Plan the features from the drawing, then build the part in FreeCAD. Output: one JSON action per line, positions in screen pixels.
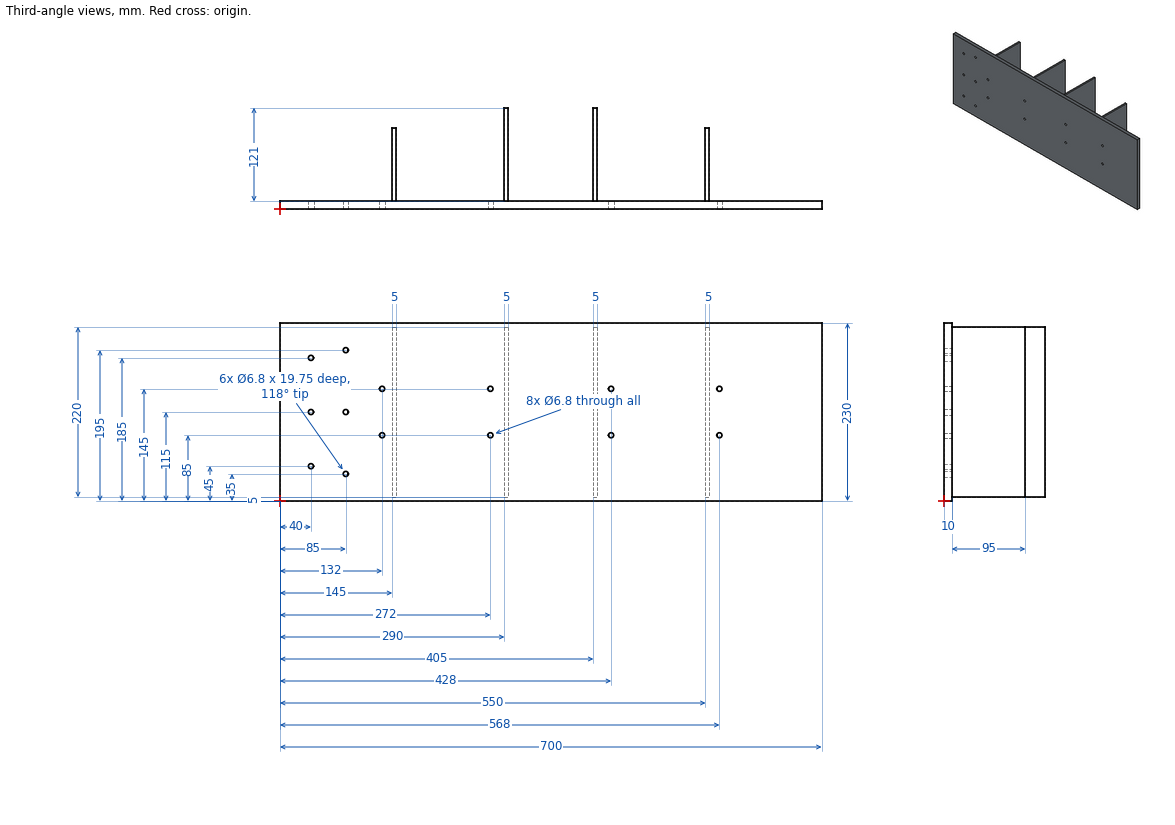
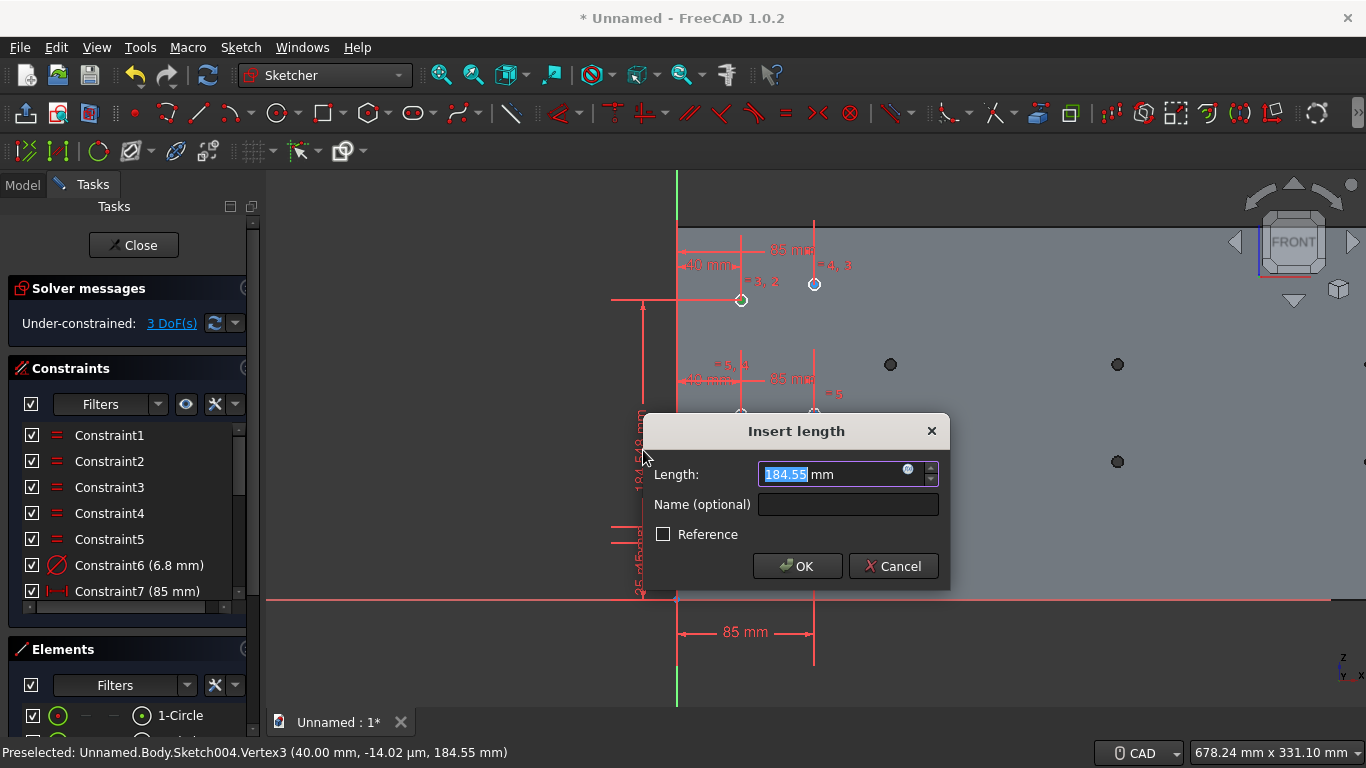
{"action": "type", "text": "185"}
{"action": "key", "text": "Return"}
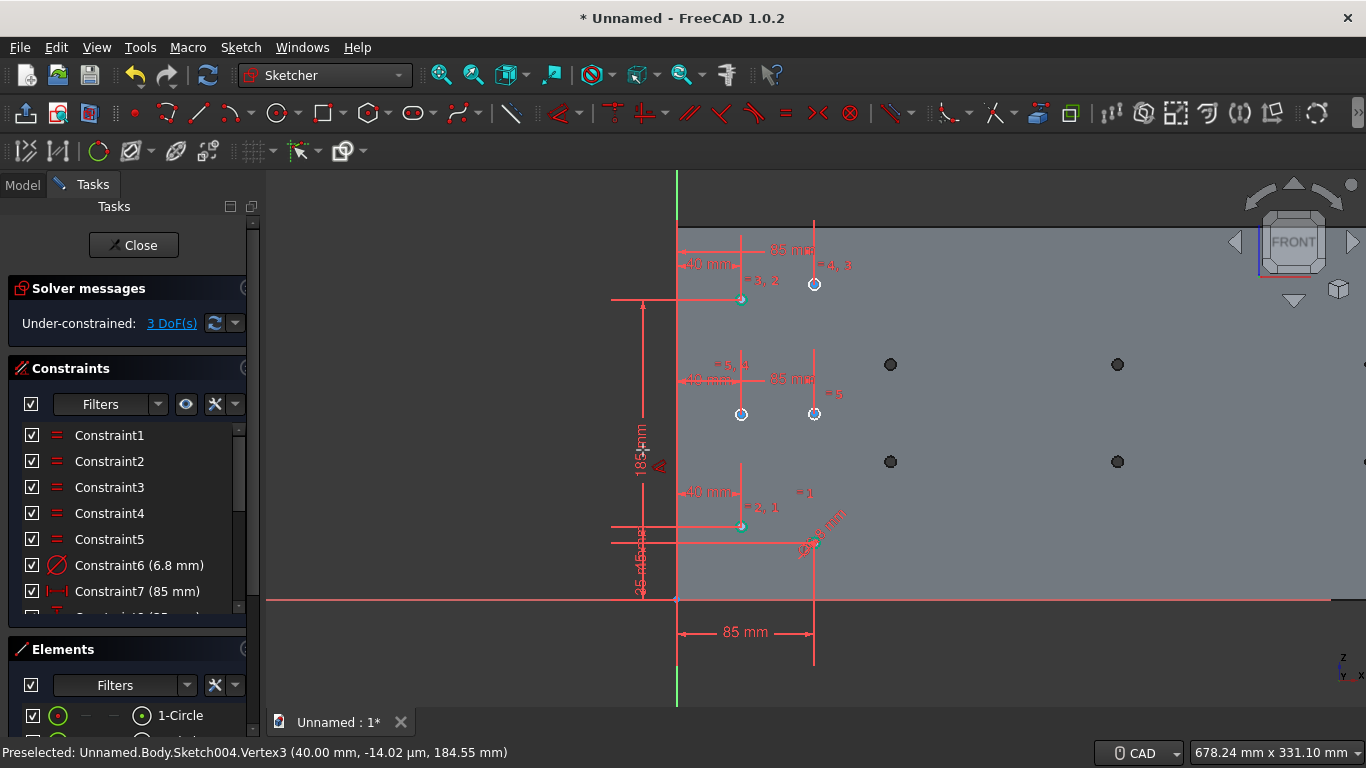
{"action": "left_click", "coordinate": [814, 285]}
{"action": "left_click", "coordinate": [643, 515]}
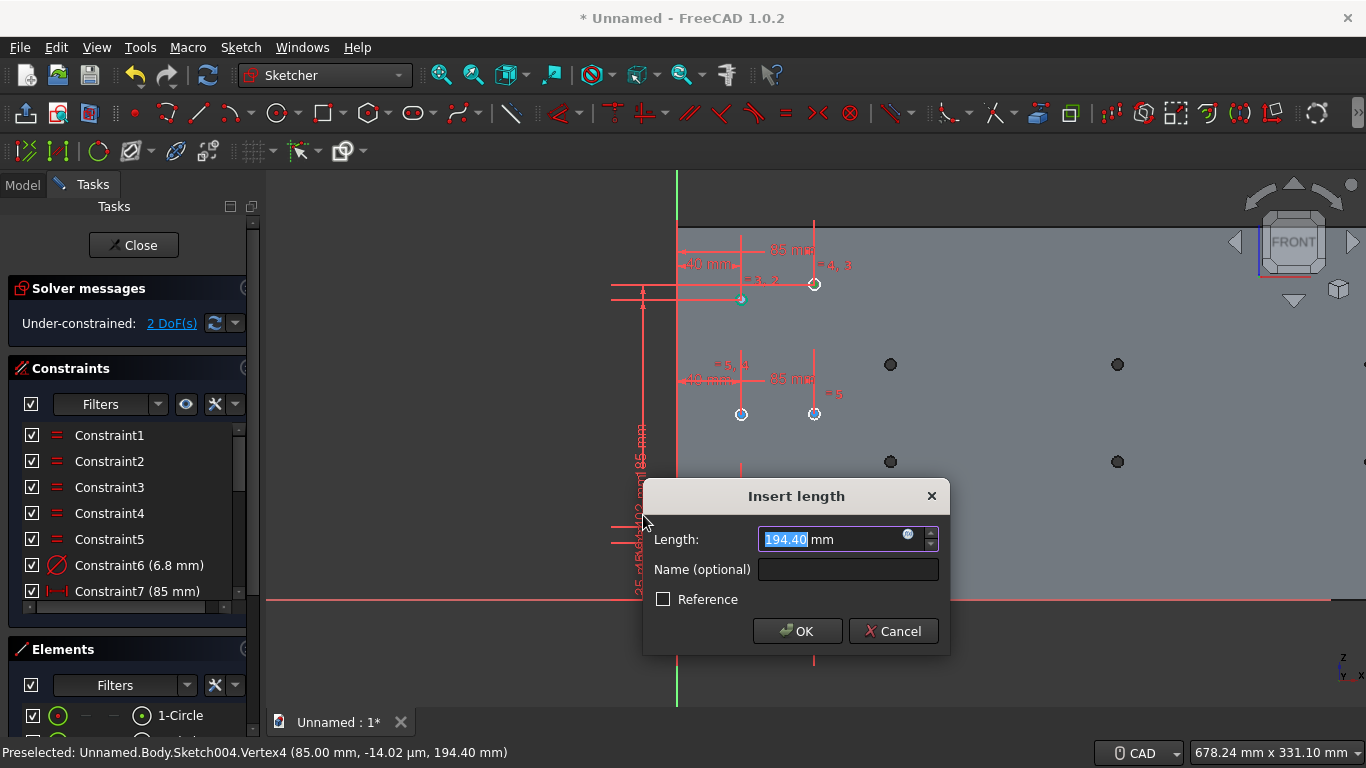
{"action": "type", "text": "195"}
{"action": "key", "text": "Return"}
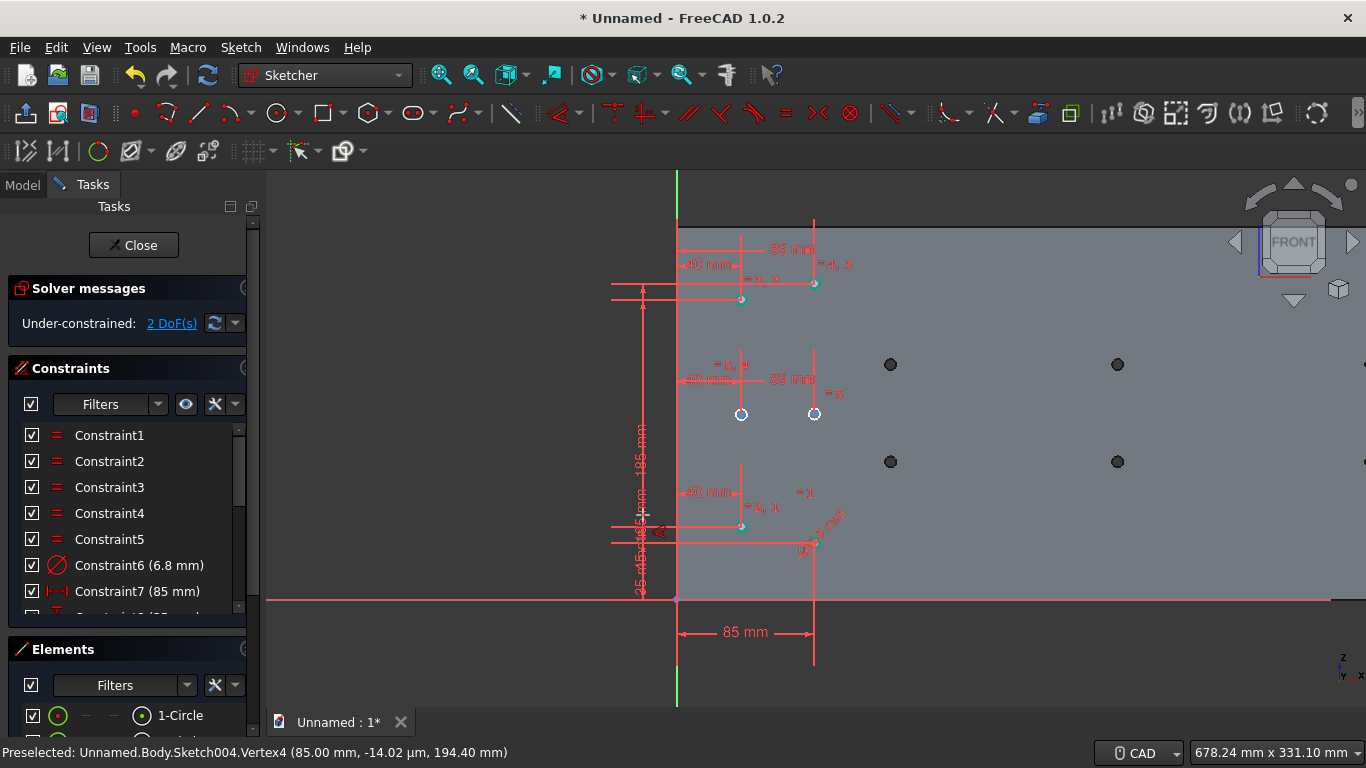
{"action": "left_click", "coordinate": [741, 415]}
{"action": "left_click", "coordinate": [775, 465]}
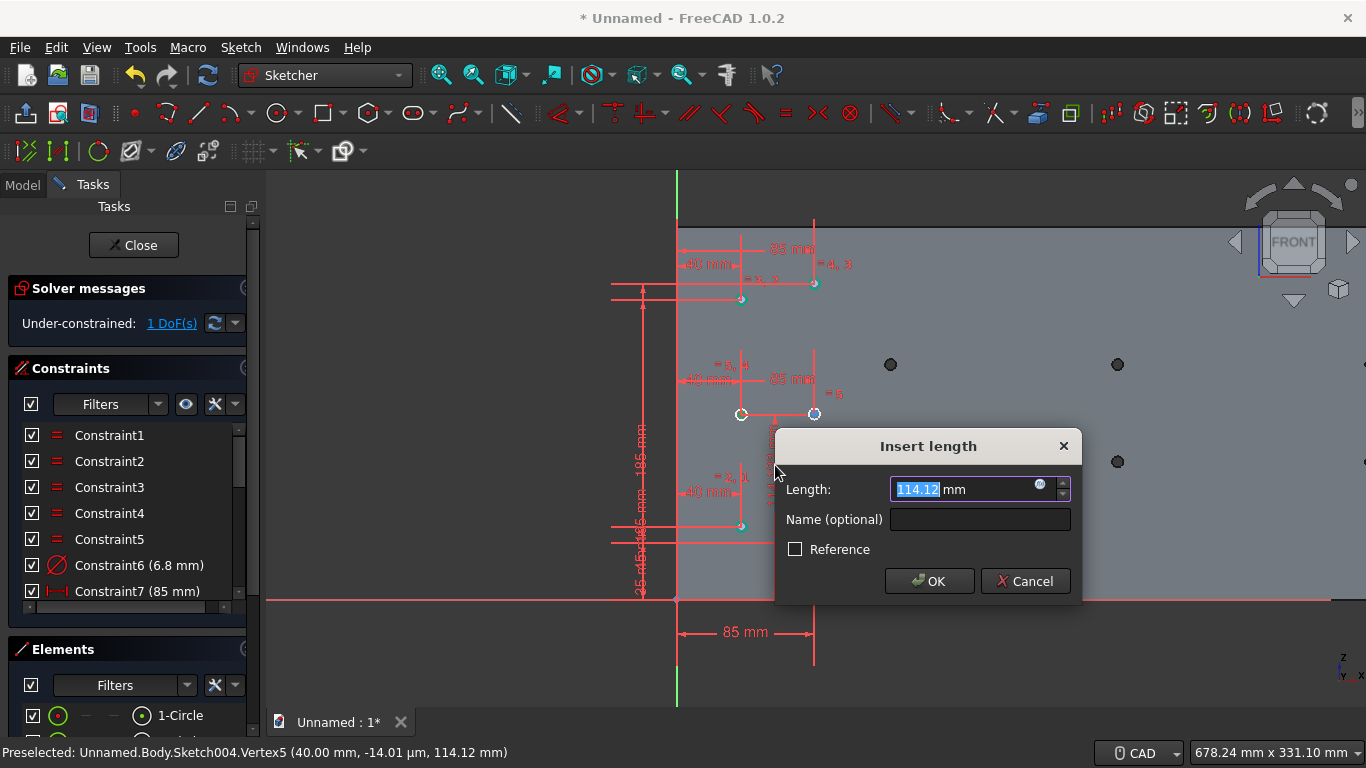
{"action": "type", "text": "115"}
{"action": "key", "text": "Return"}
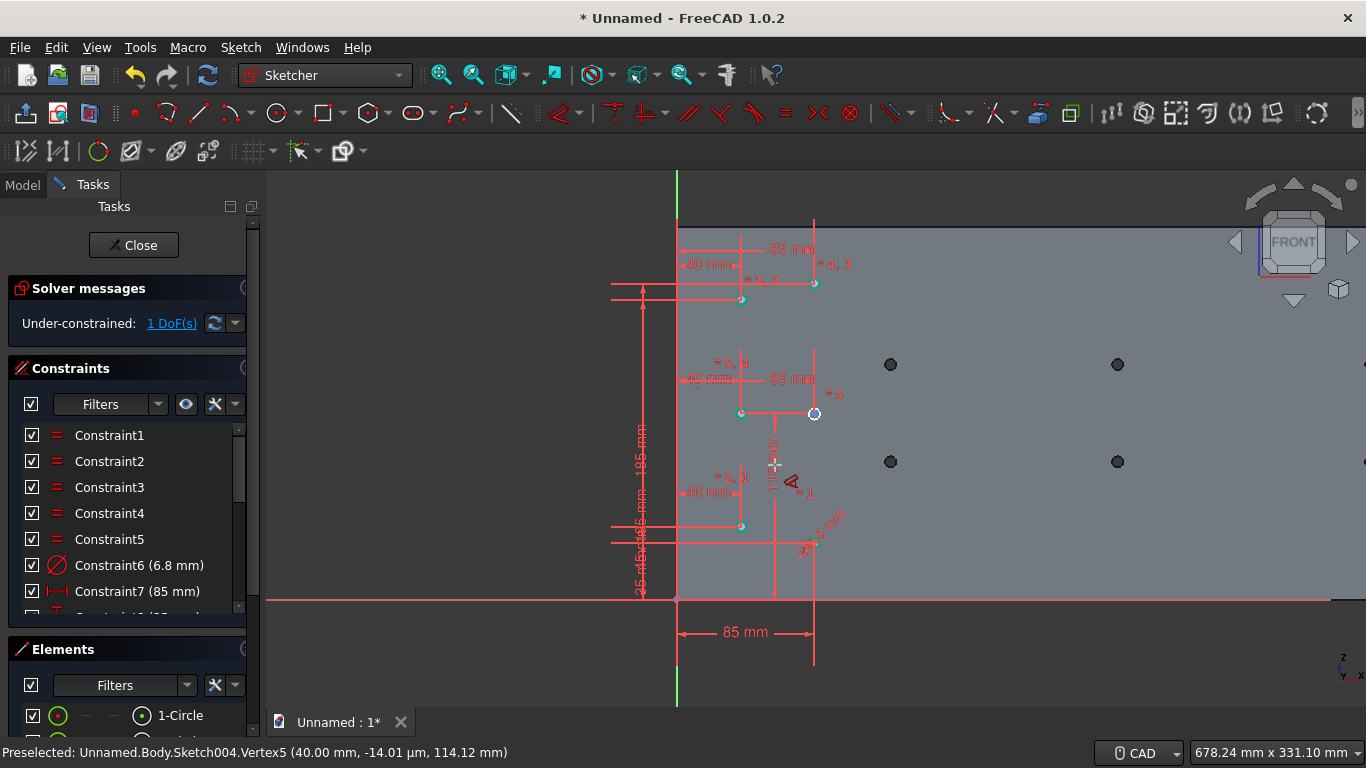
{"action": "left_click", "coordinate": [814, 414]}
{"action": "left_click", "coordinate": [848, 507]}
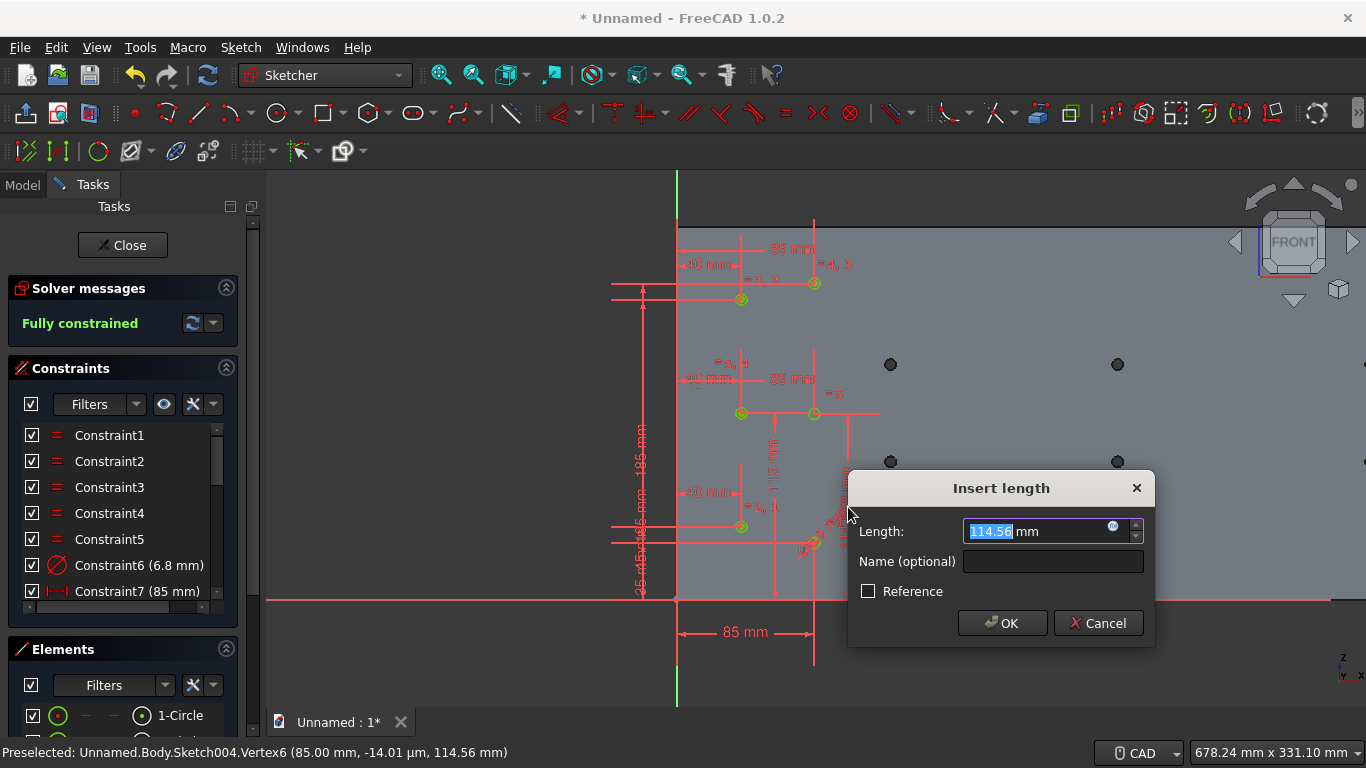
{"action": "type", "text": "115"}
{"action": "key", "text": "Return"}
{"action": "key", "text": "Escape"}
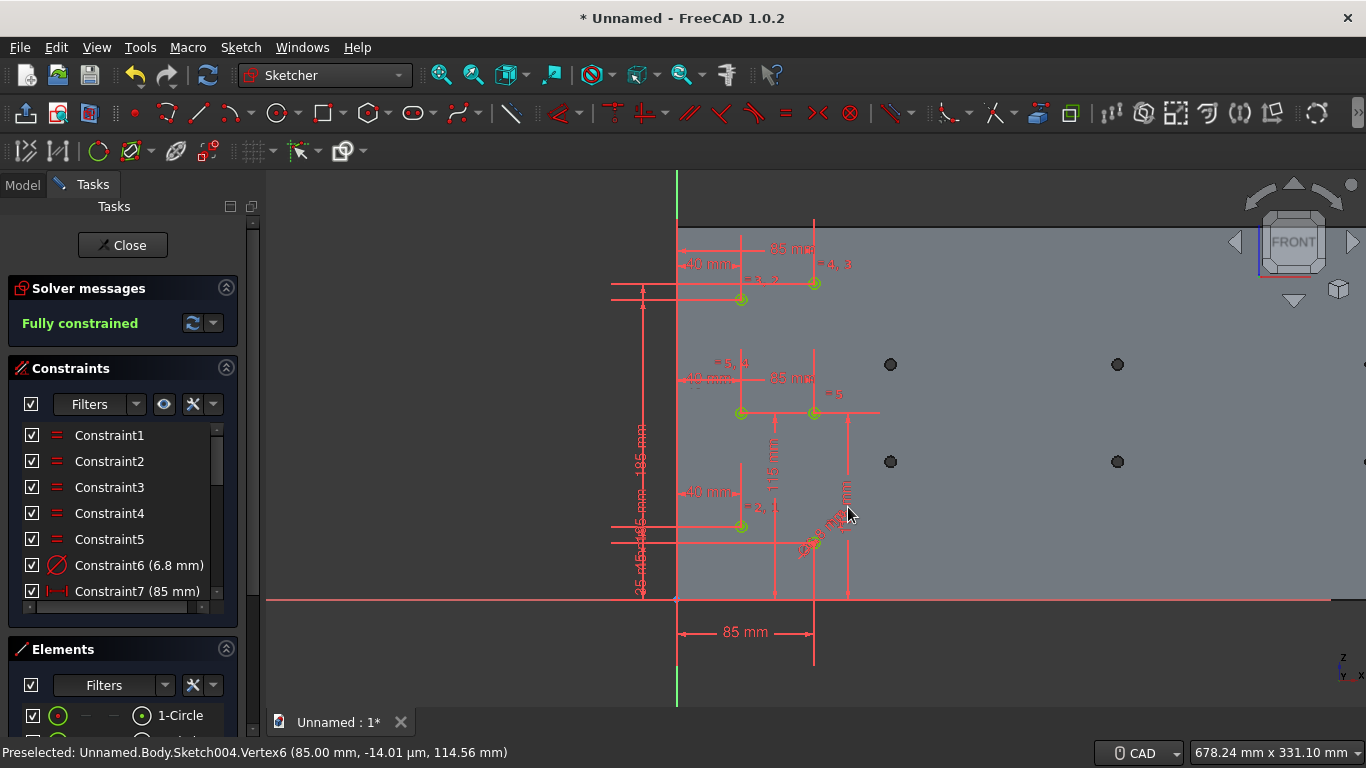
{"action": "left_click", "coordinate": [123, 245]}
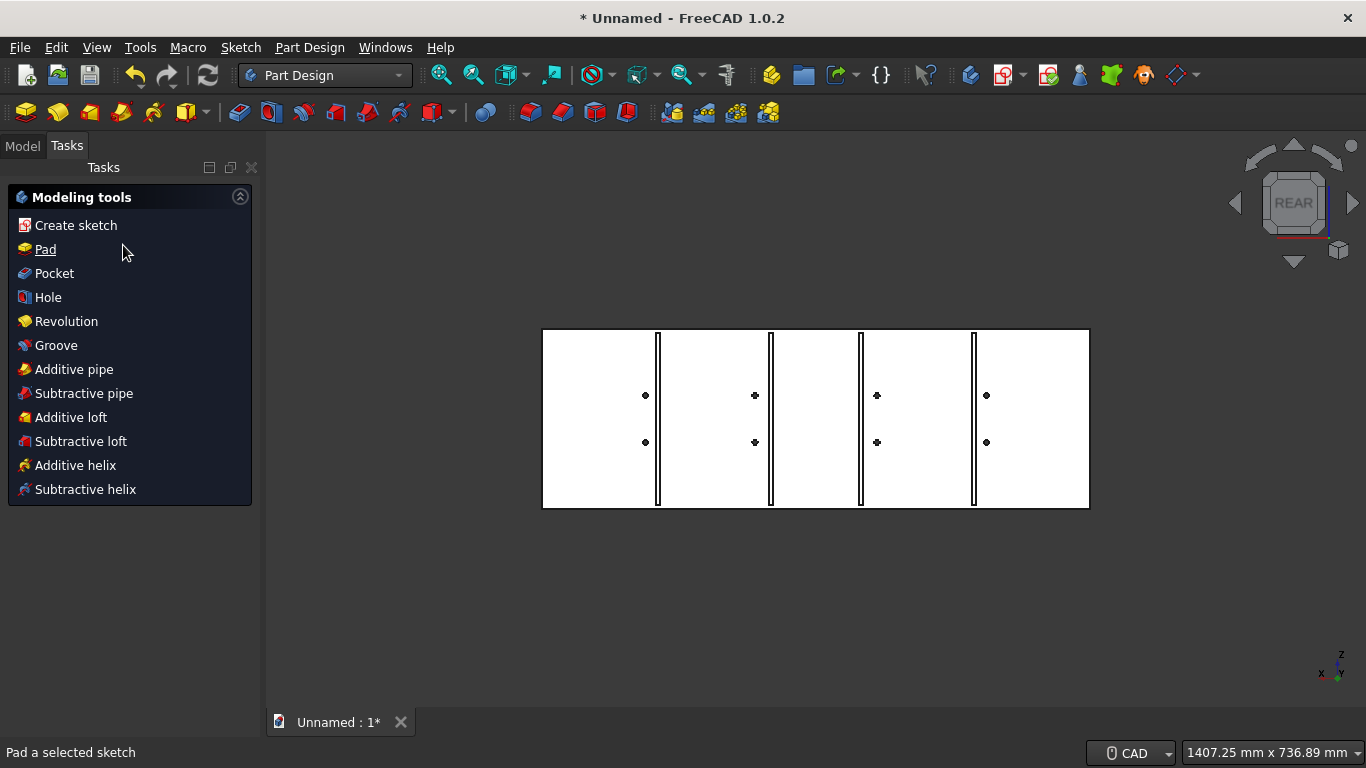
{"action": "left_click", "coordinate": [272, 112]}